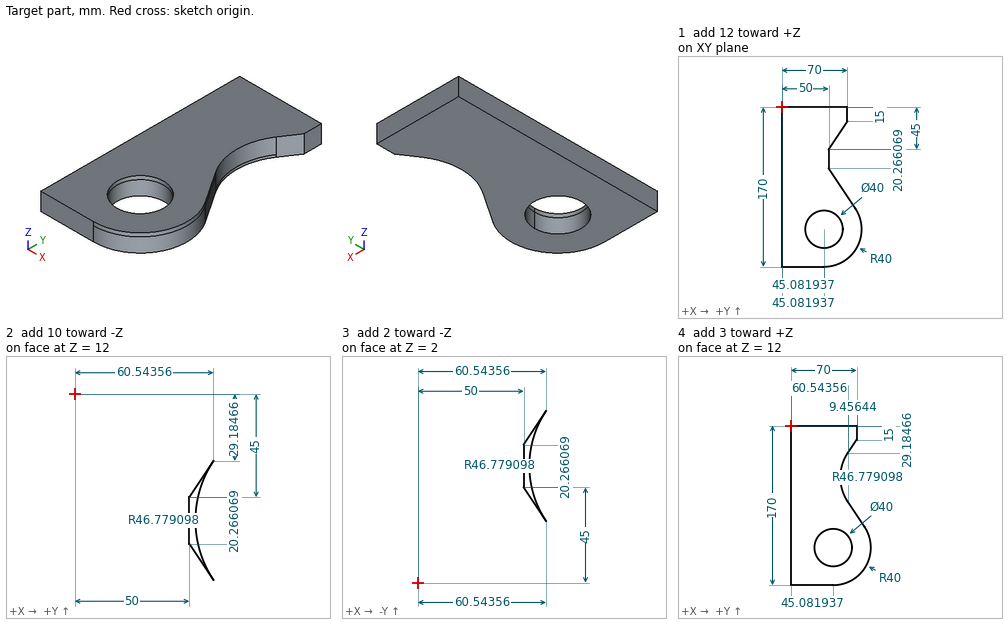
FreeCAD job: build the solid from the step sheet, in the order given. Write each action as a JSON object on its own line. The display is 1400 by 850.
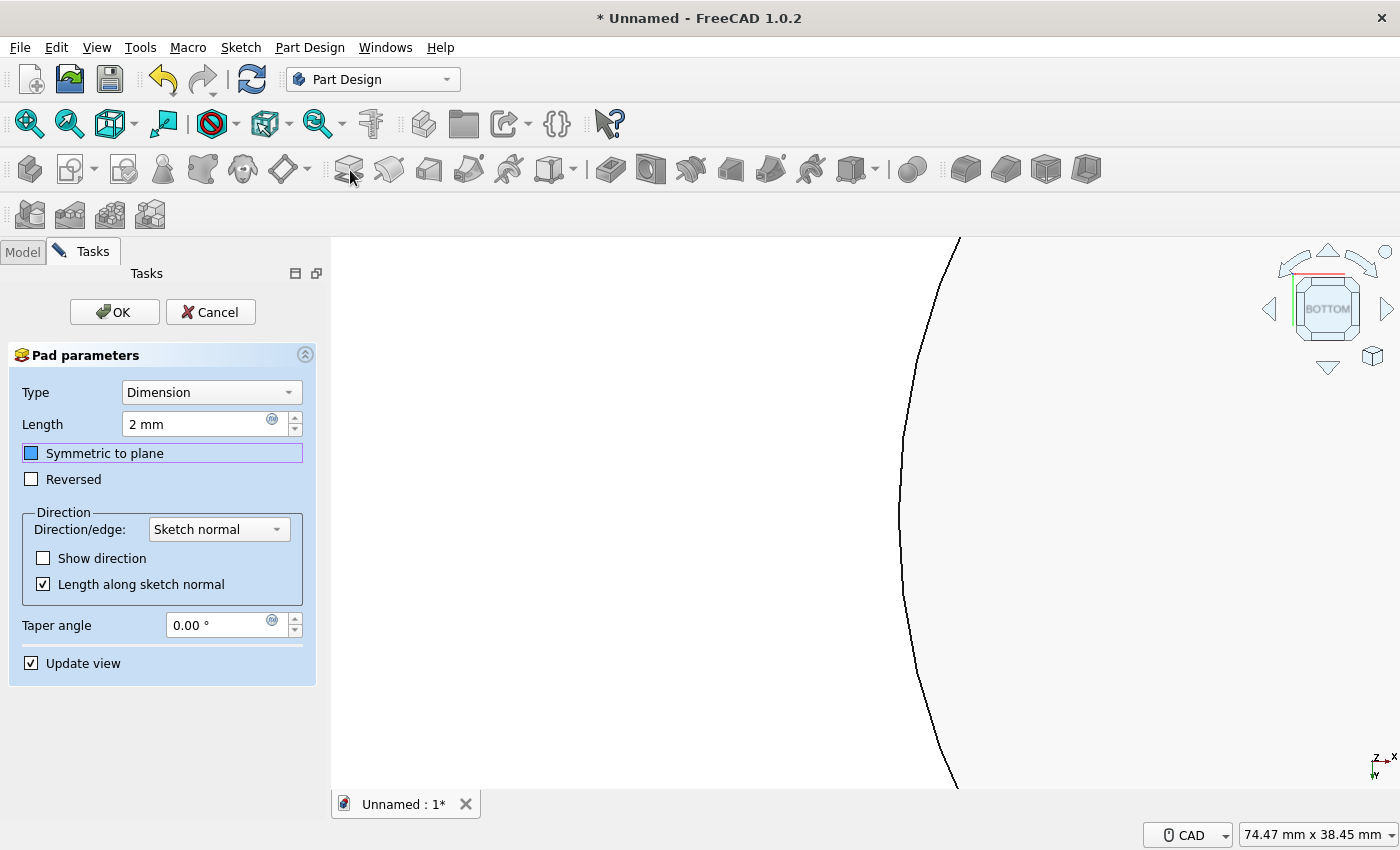
{"action": "left_click", "coordinate": [115, 312]}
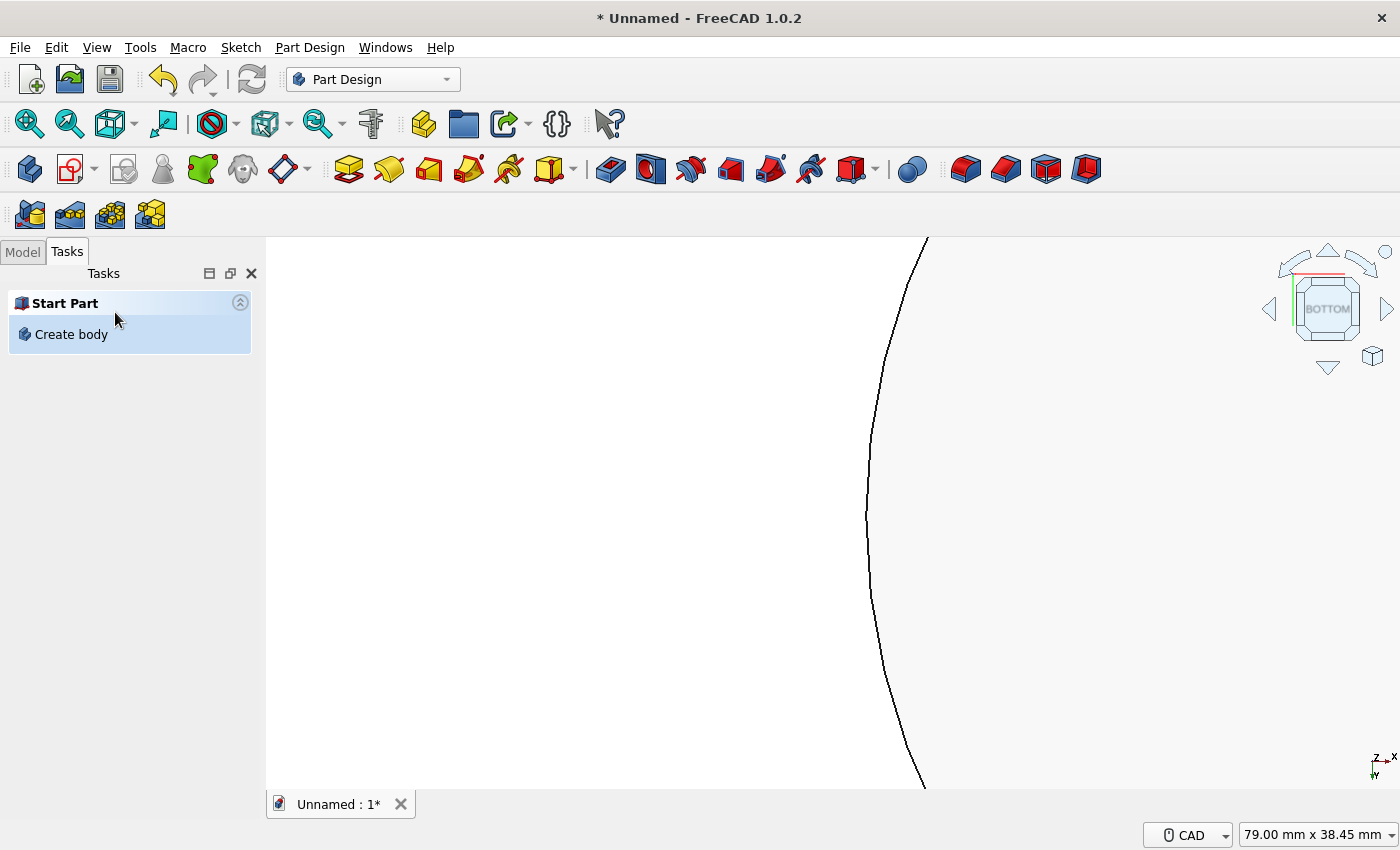
{"action": "left_click", "coordinate": [30, 124]}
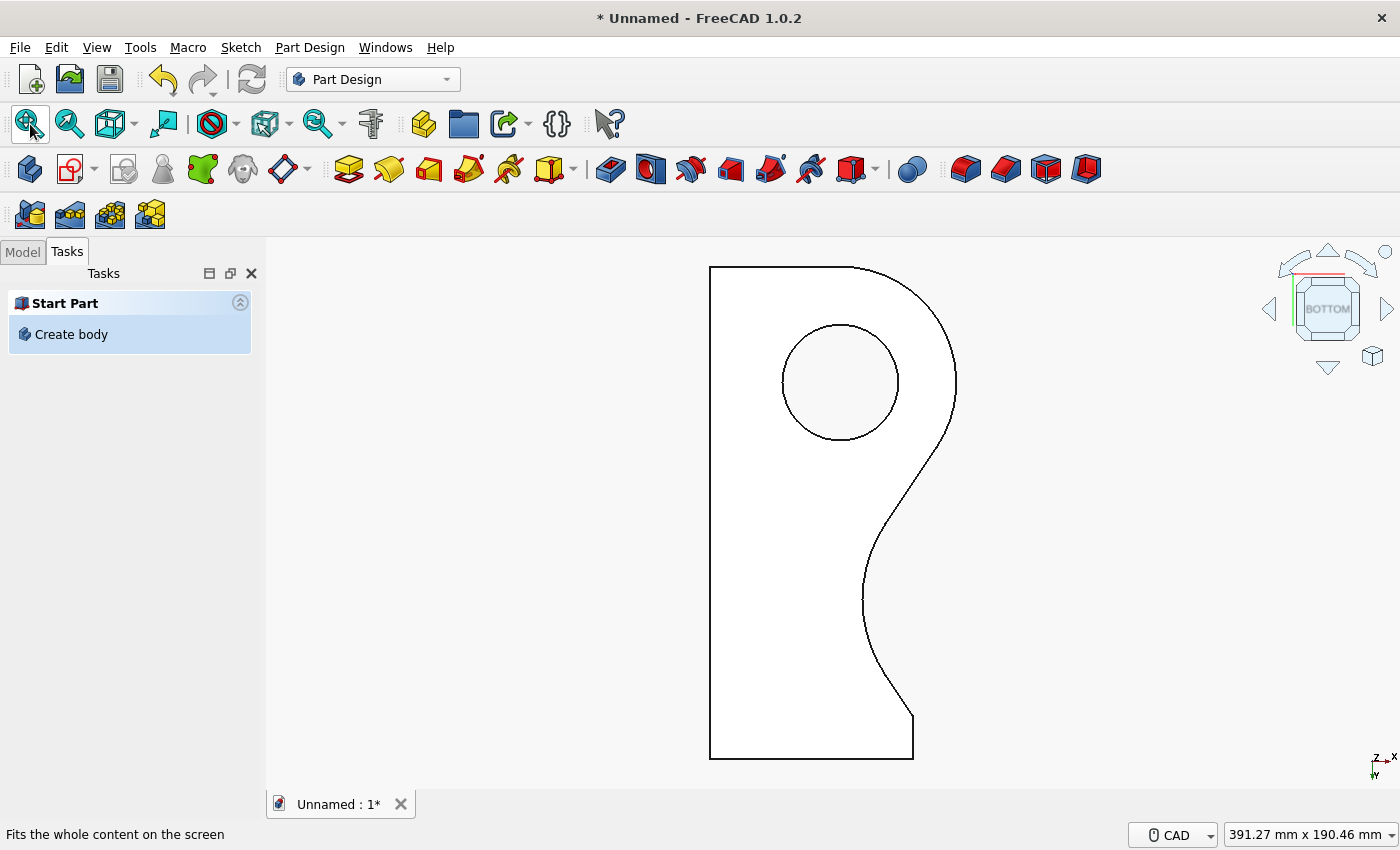
{"action": "key", "text": "0"}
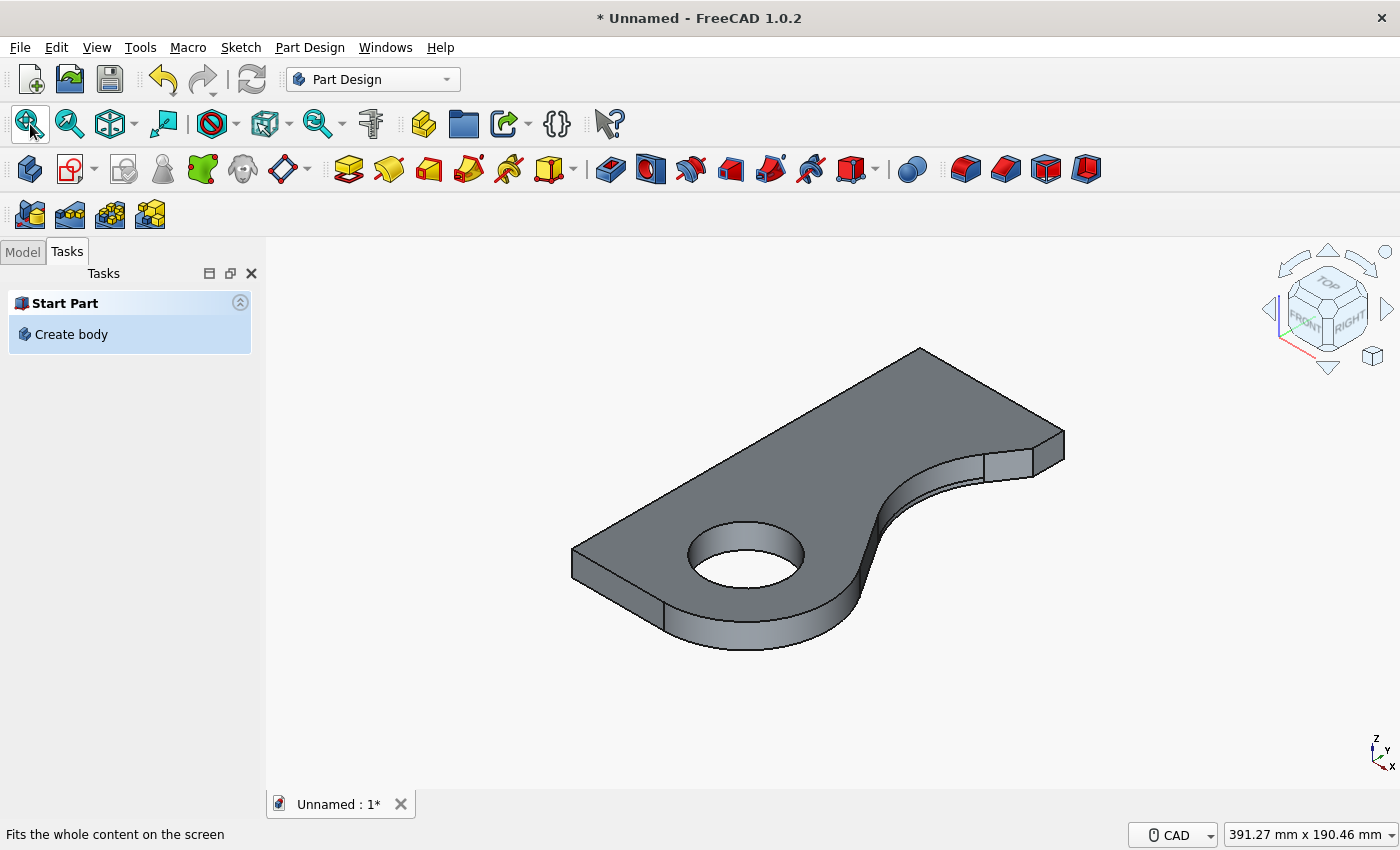
{"action": "left_click", "coordinate": [808, 483]}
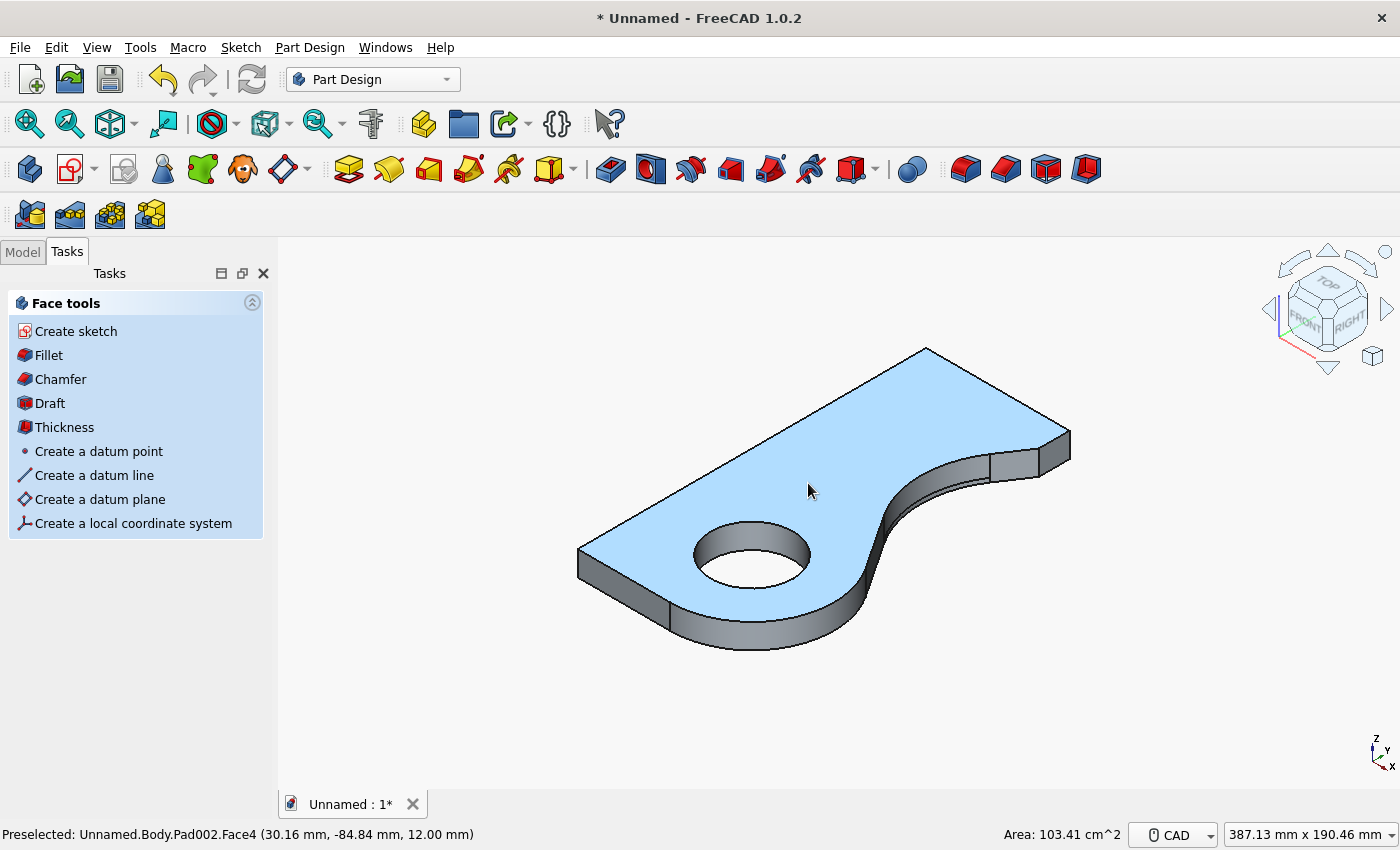
{"action": "left_click", "coordinate": [70, 170]}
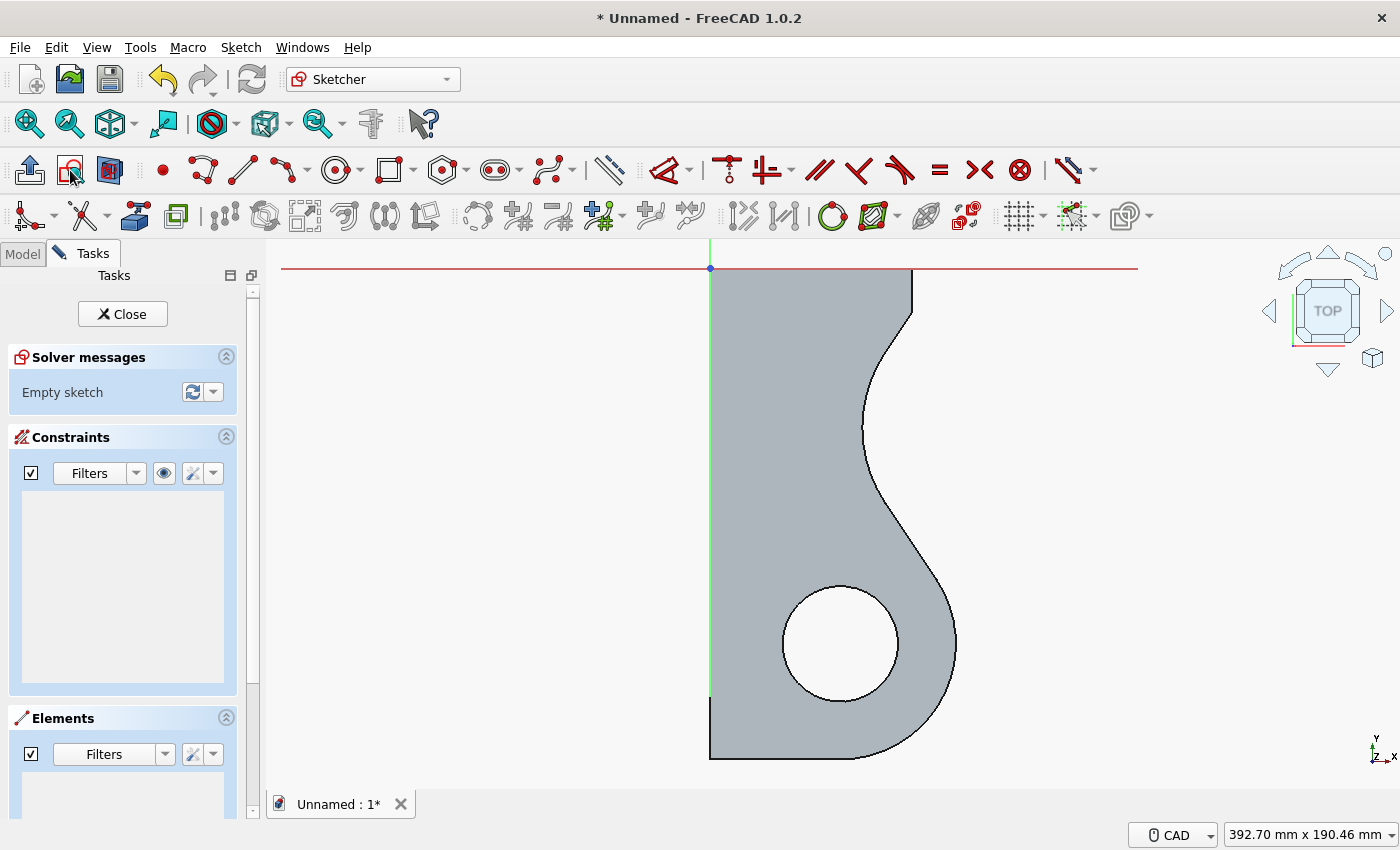
{"action": "scroll", "coordinate": [639, 514], "scroll_direction": "down", "scroll_amount": 2}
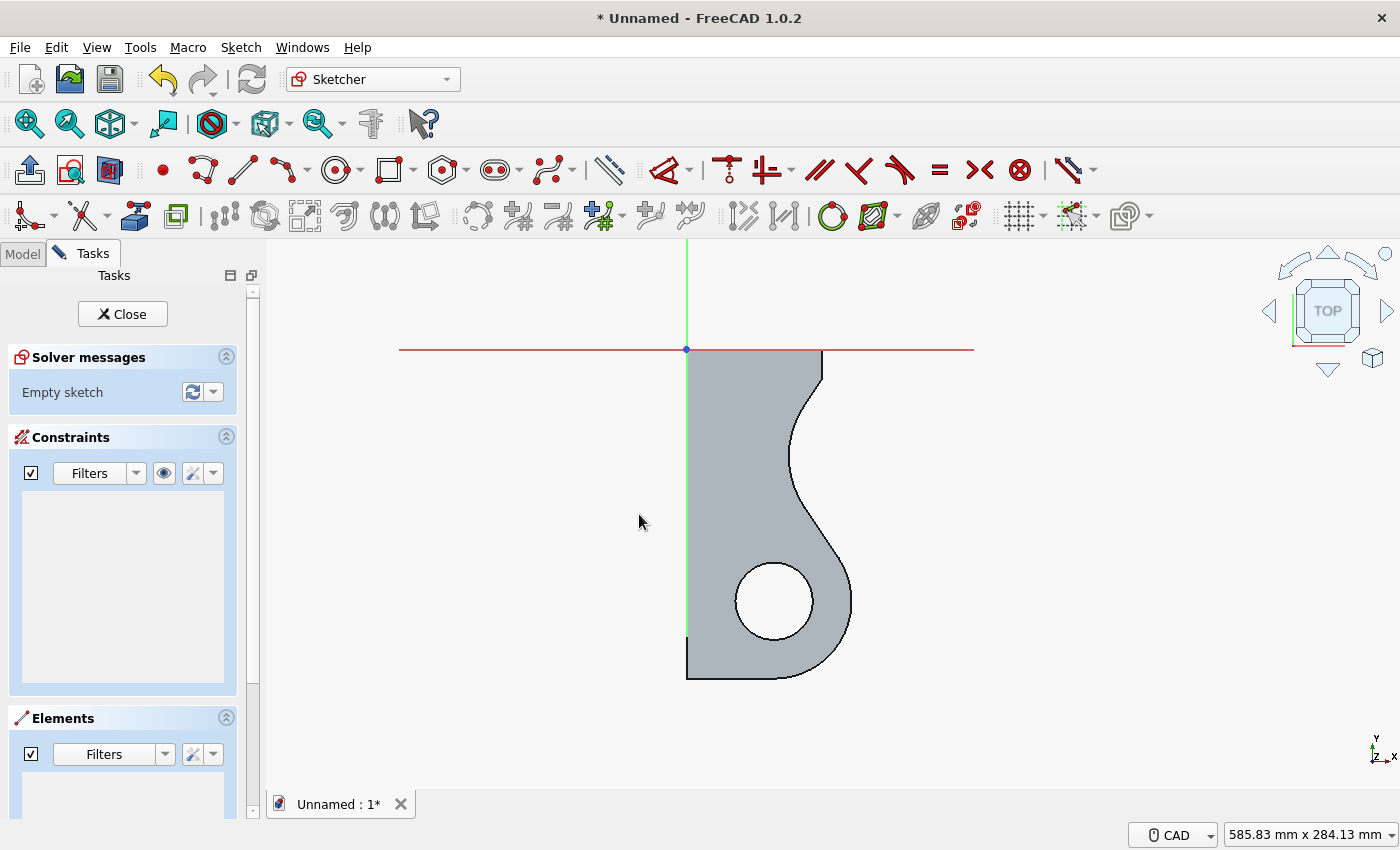
{"action": "left_click", "coordinate": [244, 170]}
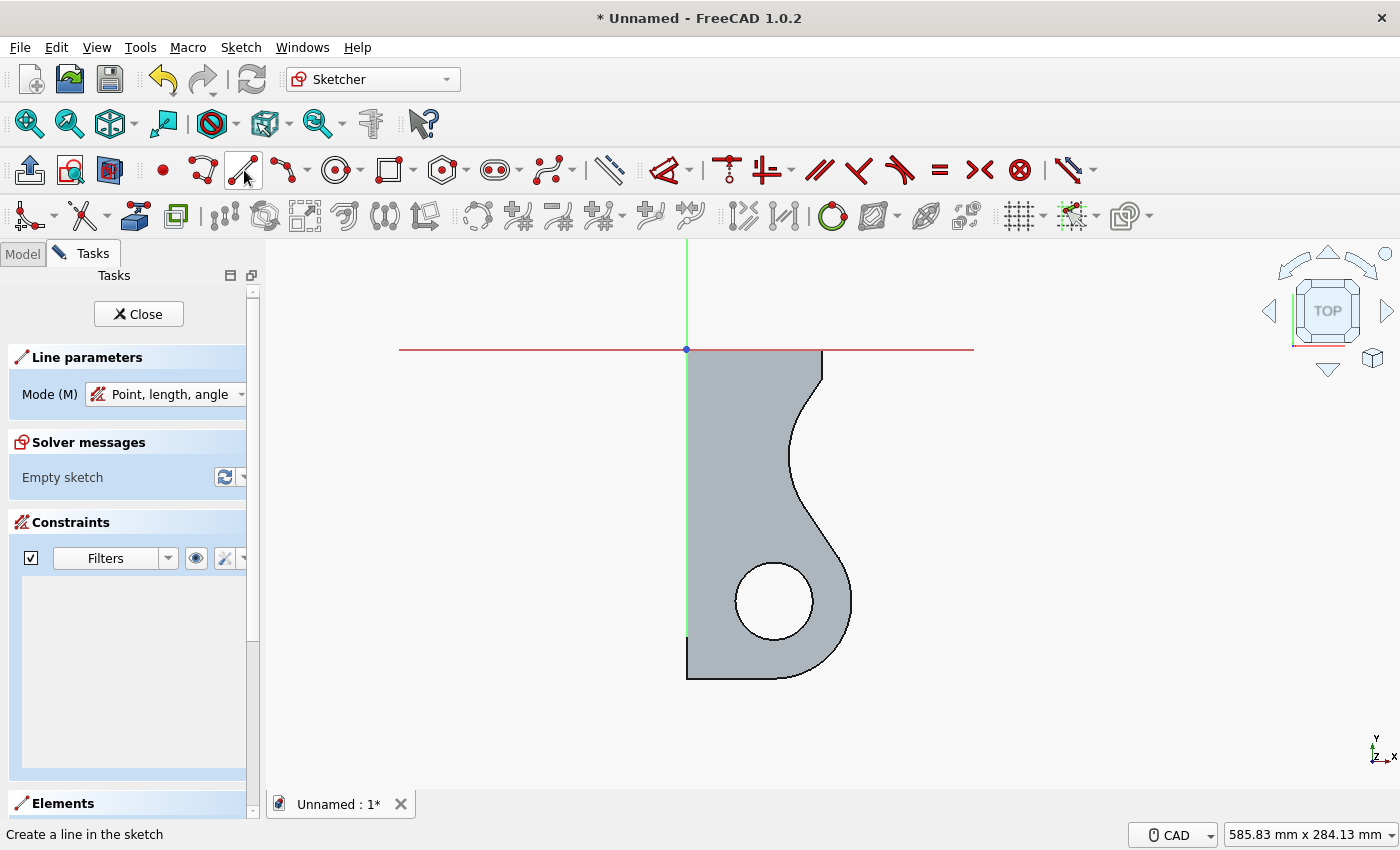
{"action": "left_click", "coordinate": [839, 558]}
{"action": "left_click", "coordinate": [804, 507]}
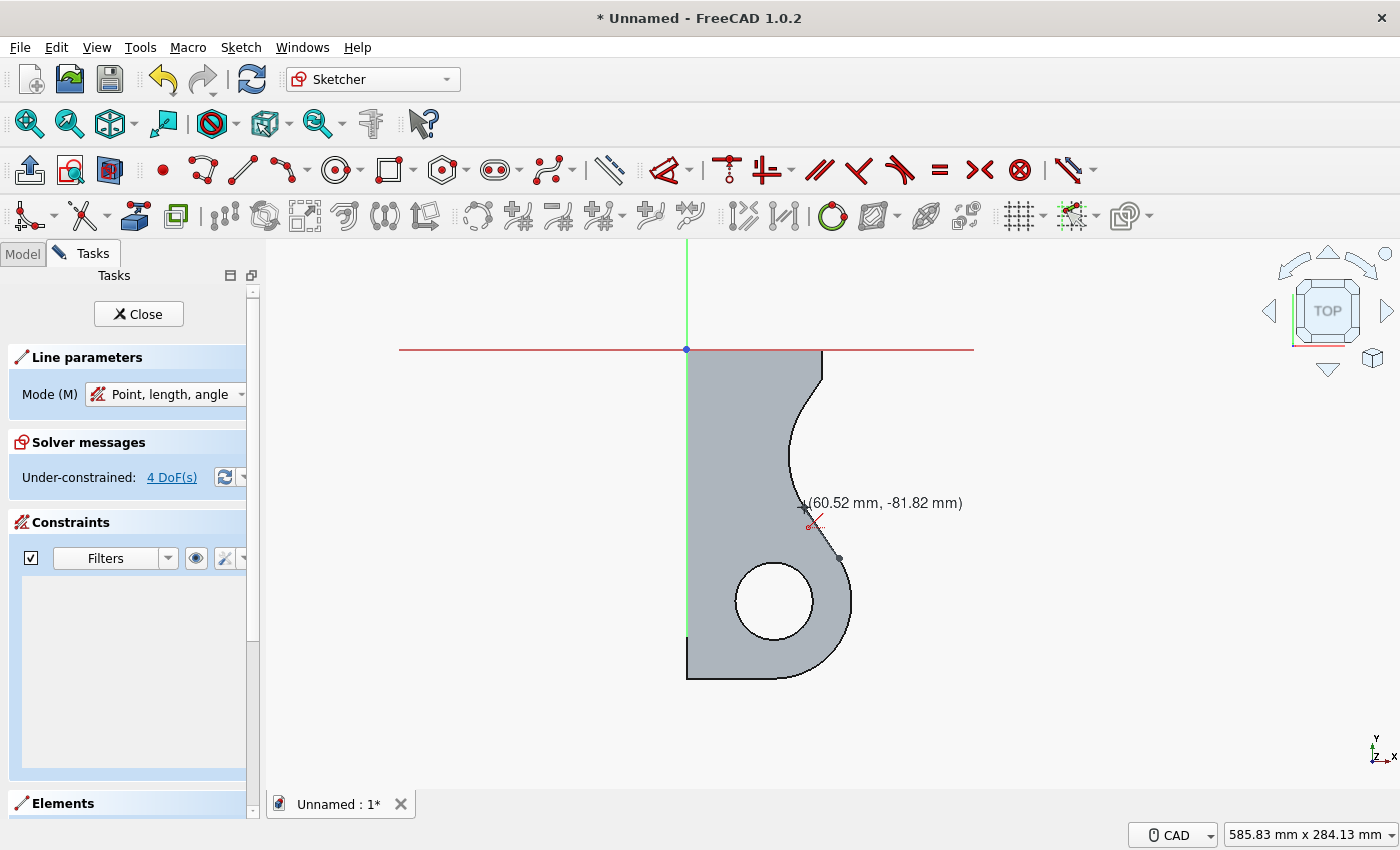
{"action": "left_click", "coordinate": [204, 170]}